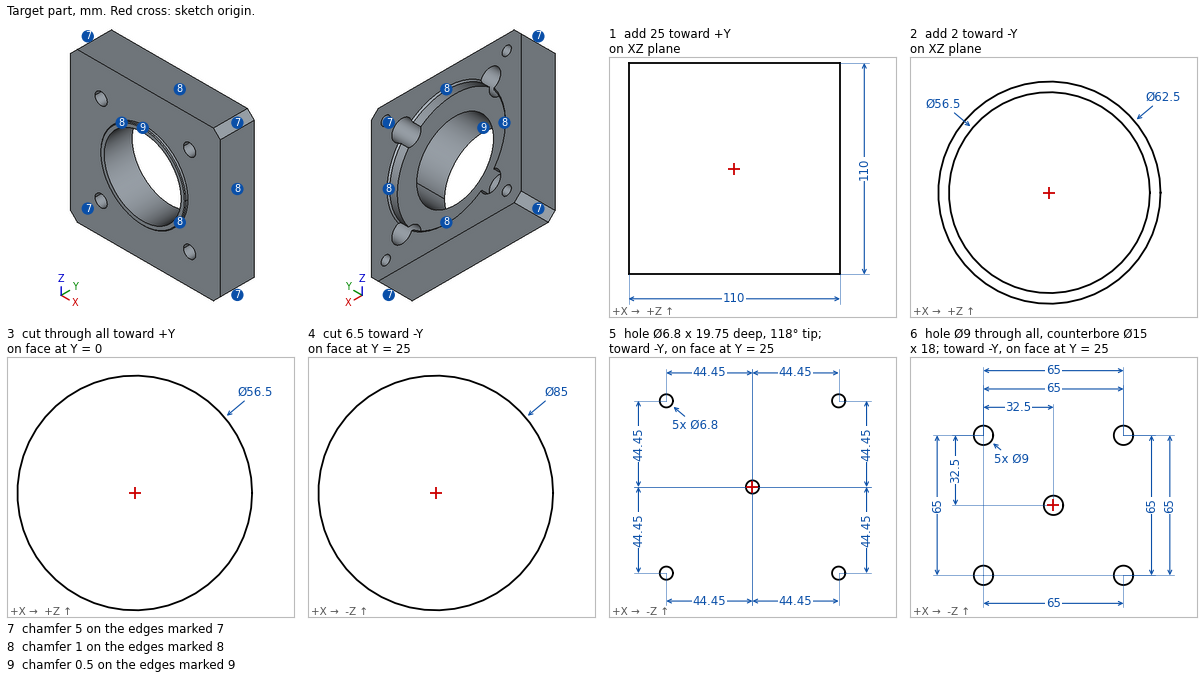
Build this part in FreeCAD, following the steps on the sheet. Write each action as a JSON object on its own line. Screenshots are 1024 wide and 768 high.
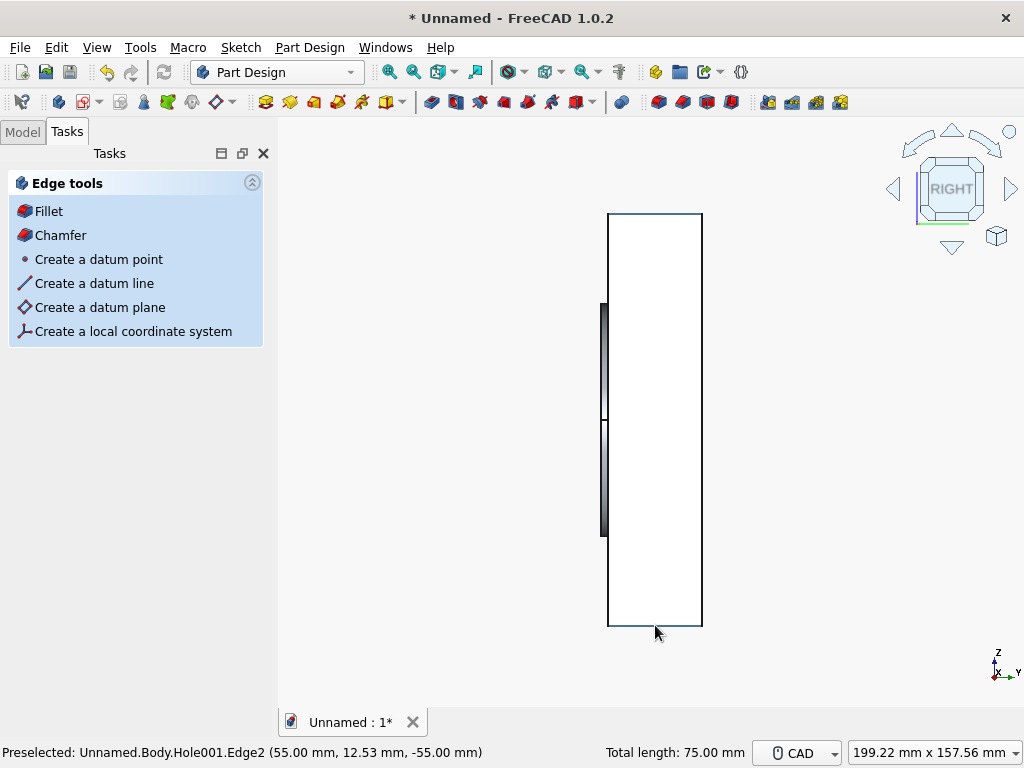
{"action": "key", "text": "5"}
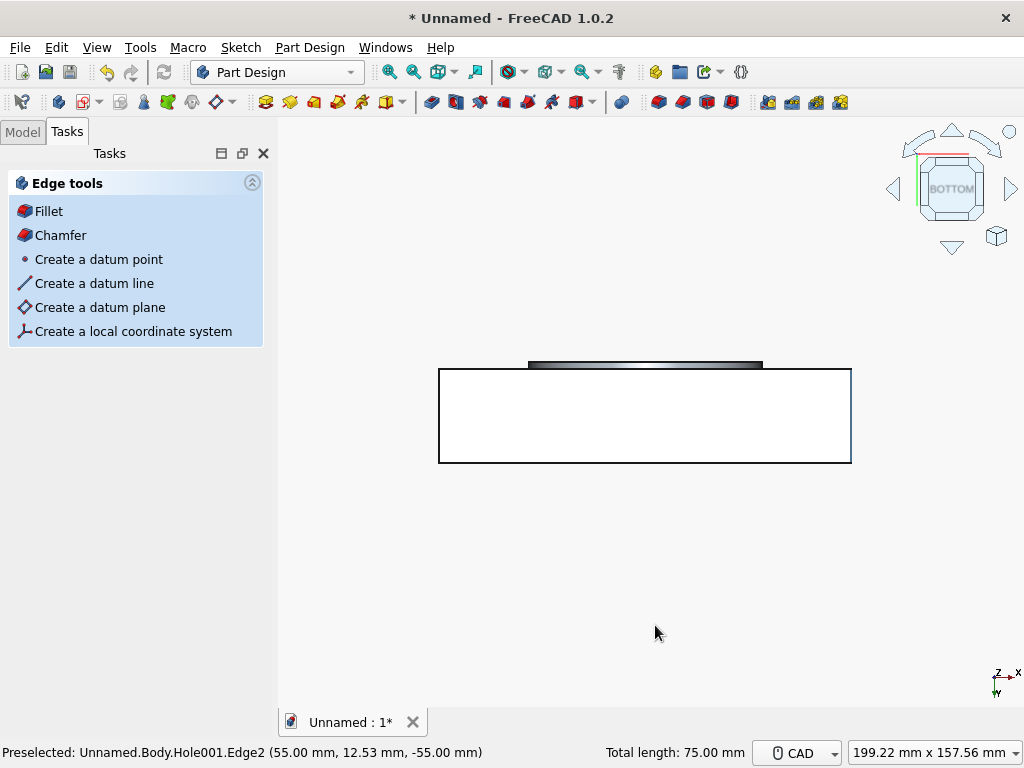
{"action": "left_click", "coordinate": [439, 415], "text": "ctrl"}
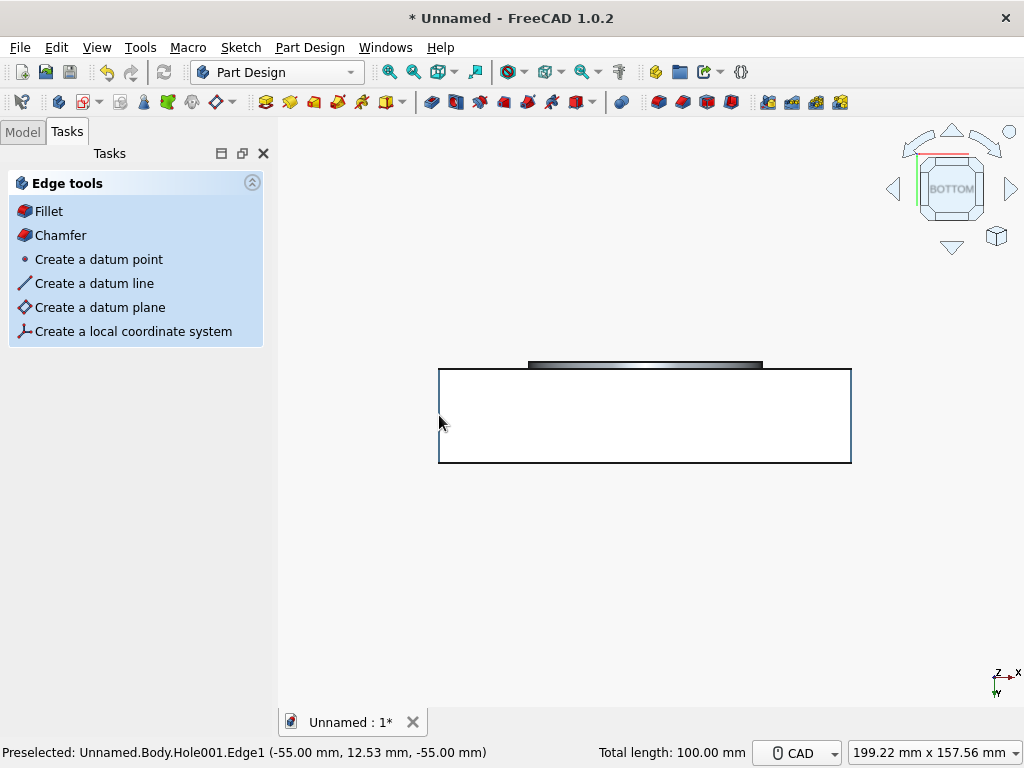
{"action": "left_click", "coordinate": [684, 102]}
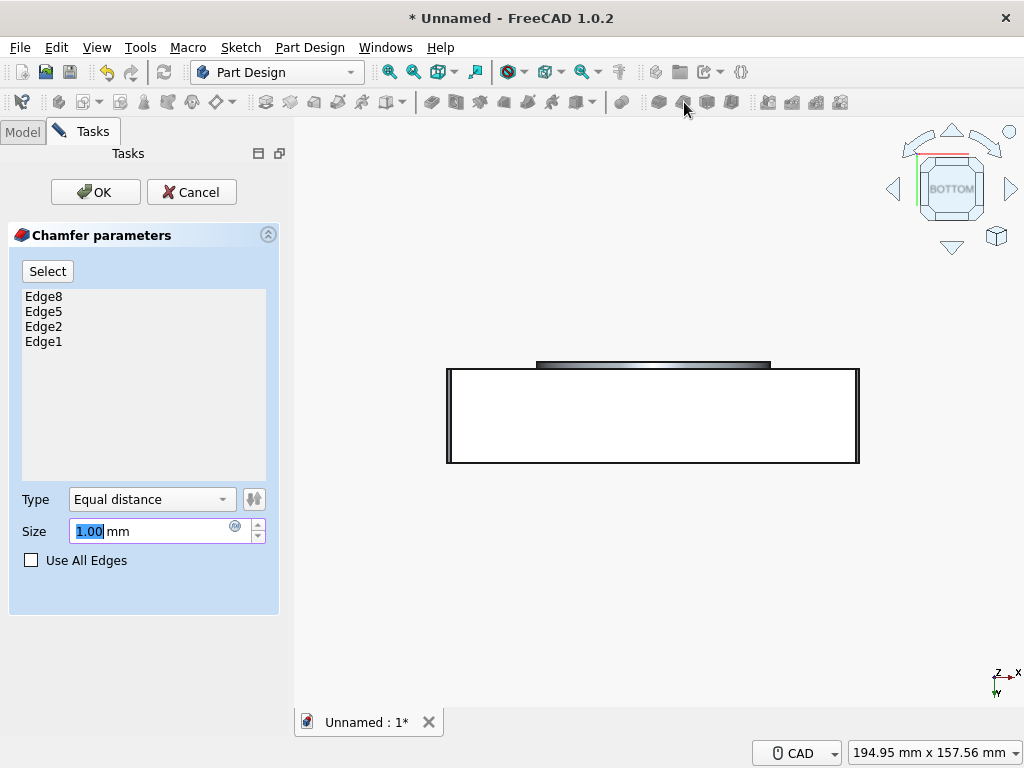
{"action": "type", "text": "5"}
{"action": "key", "text": "Tab"}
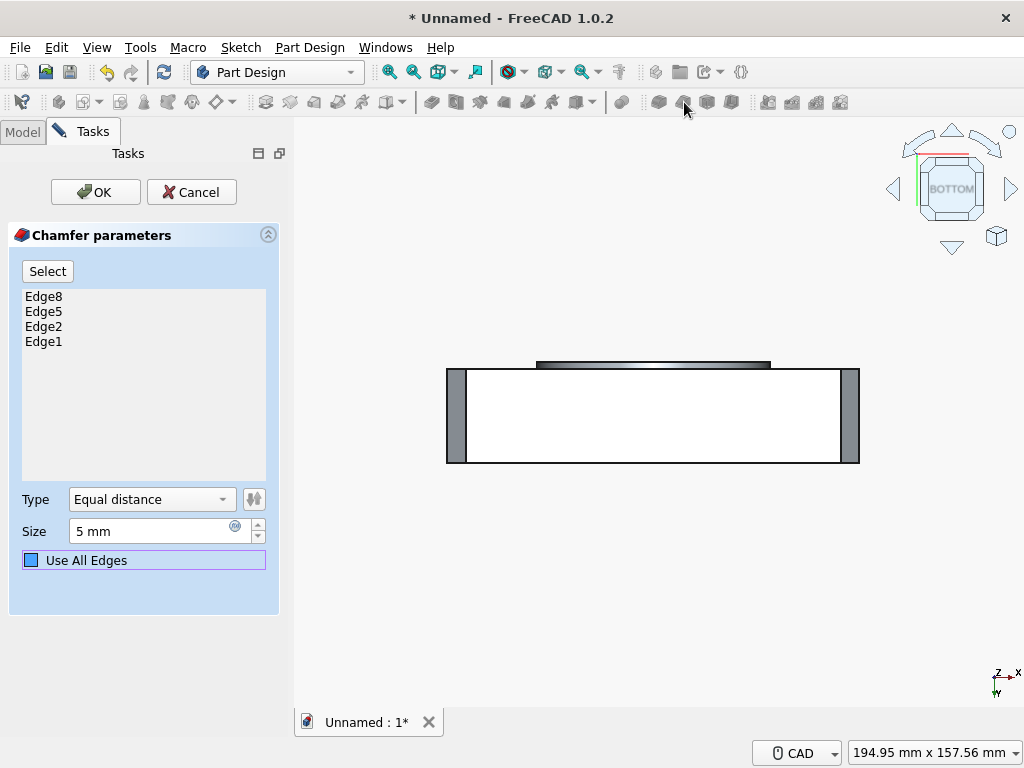
{"action": "left_click", "coordinate": [96, 192]}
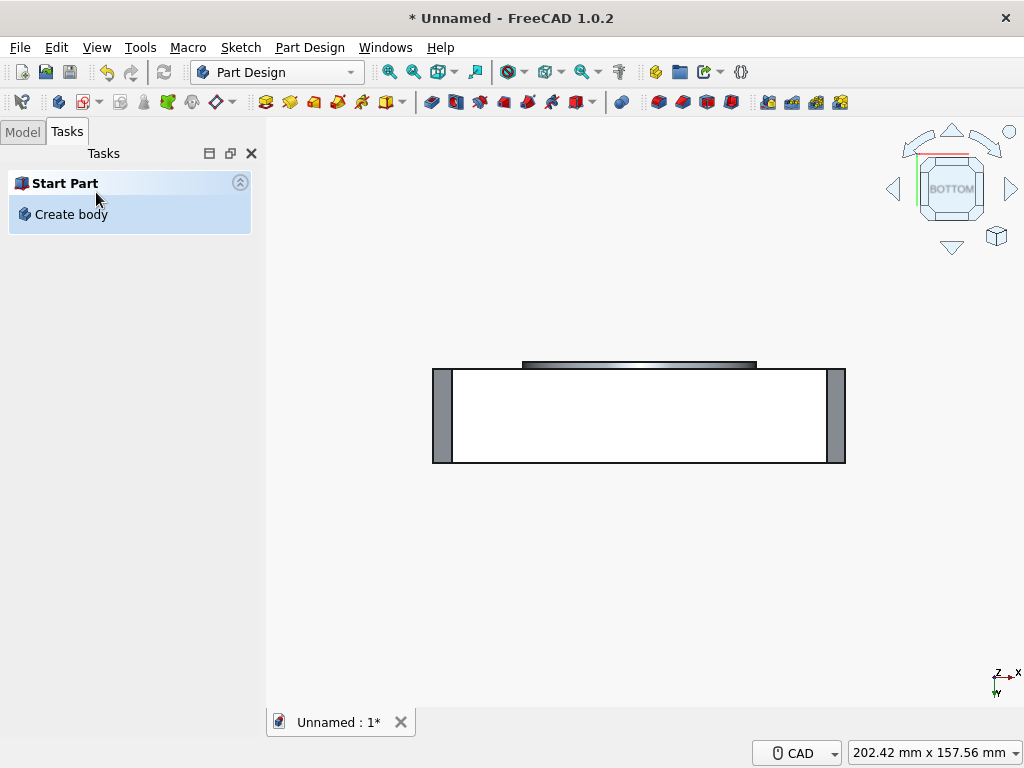
{"action": "key", "text": "0"}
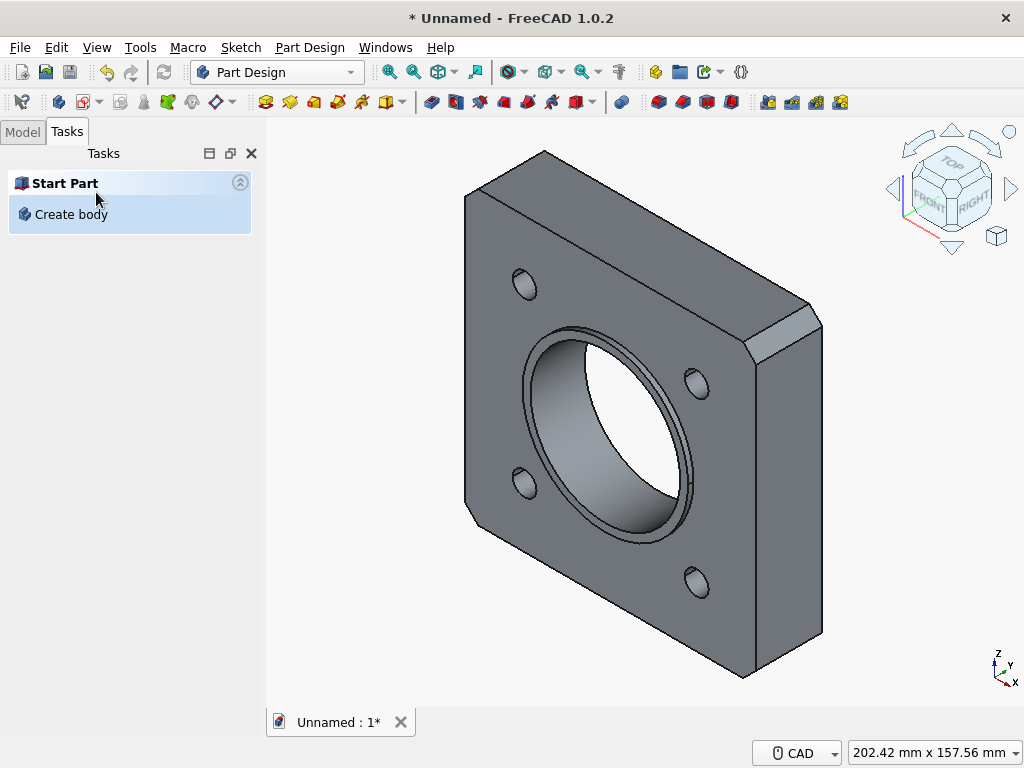
{"action": "key", "text": "2"}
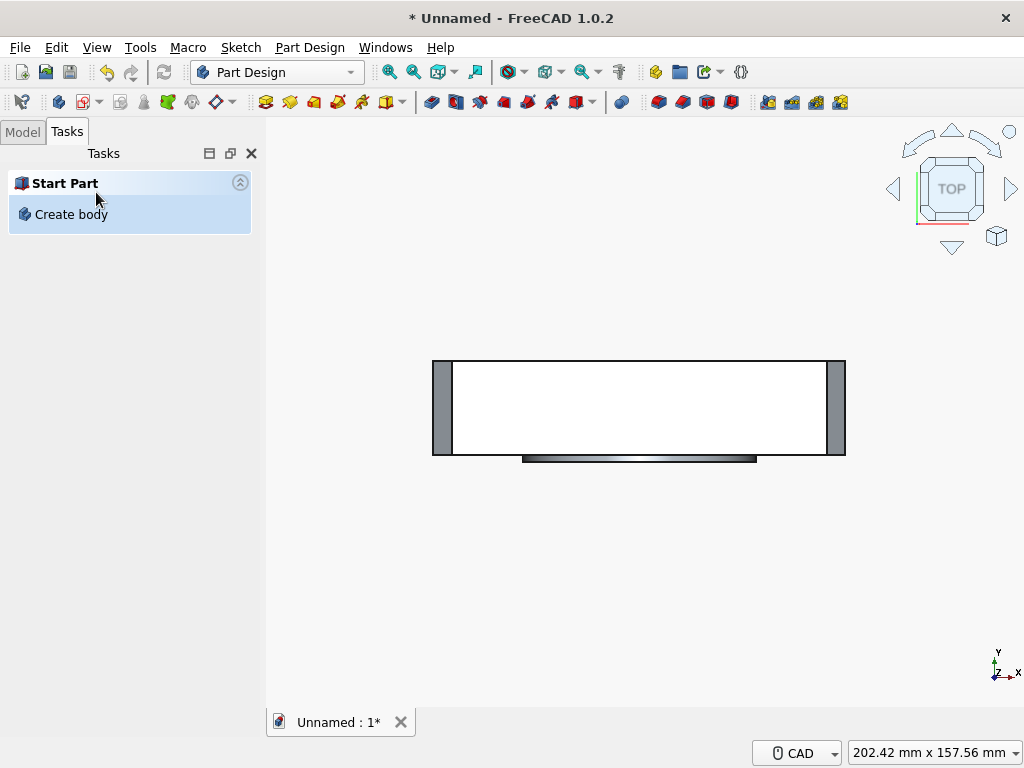
{"action": "key", "text": "1"}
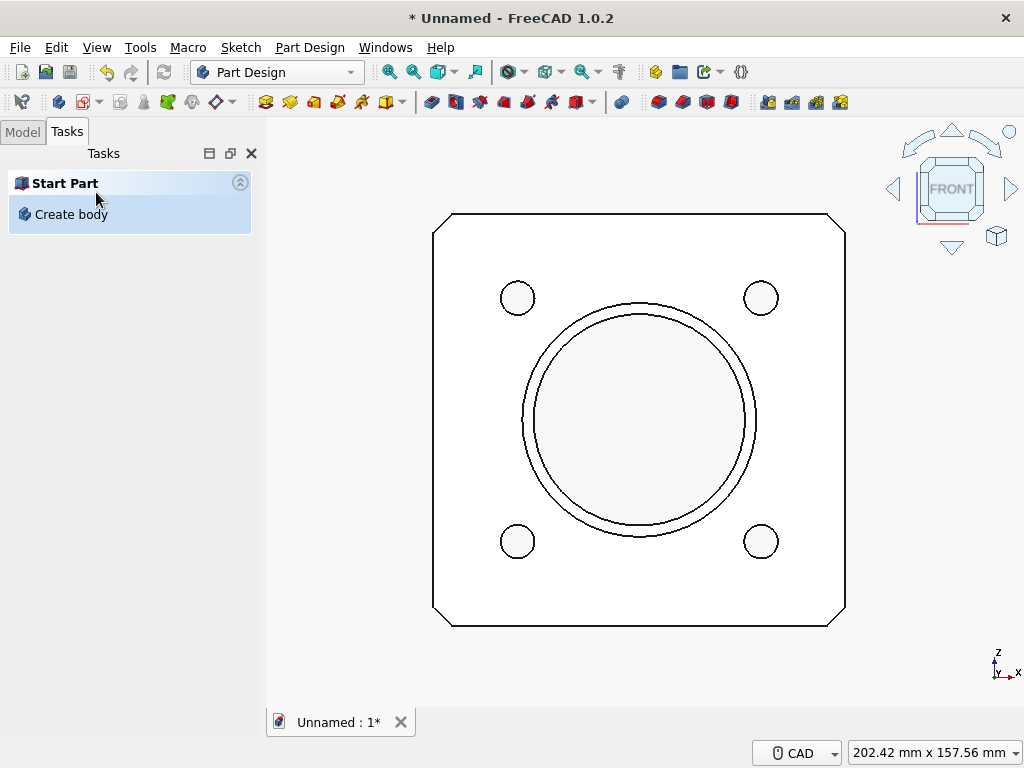
{"action": "key", "text": "3"}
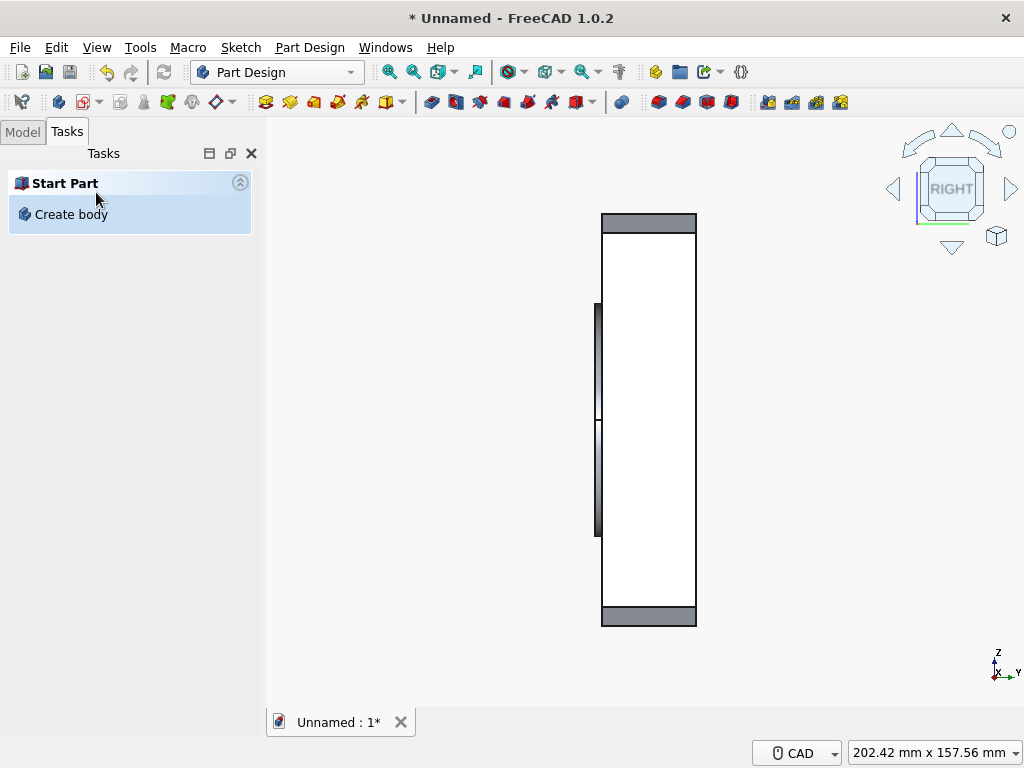
{"action": "key", "text": "5"}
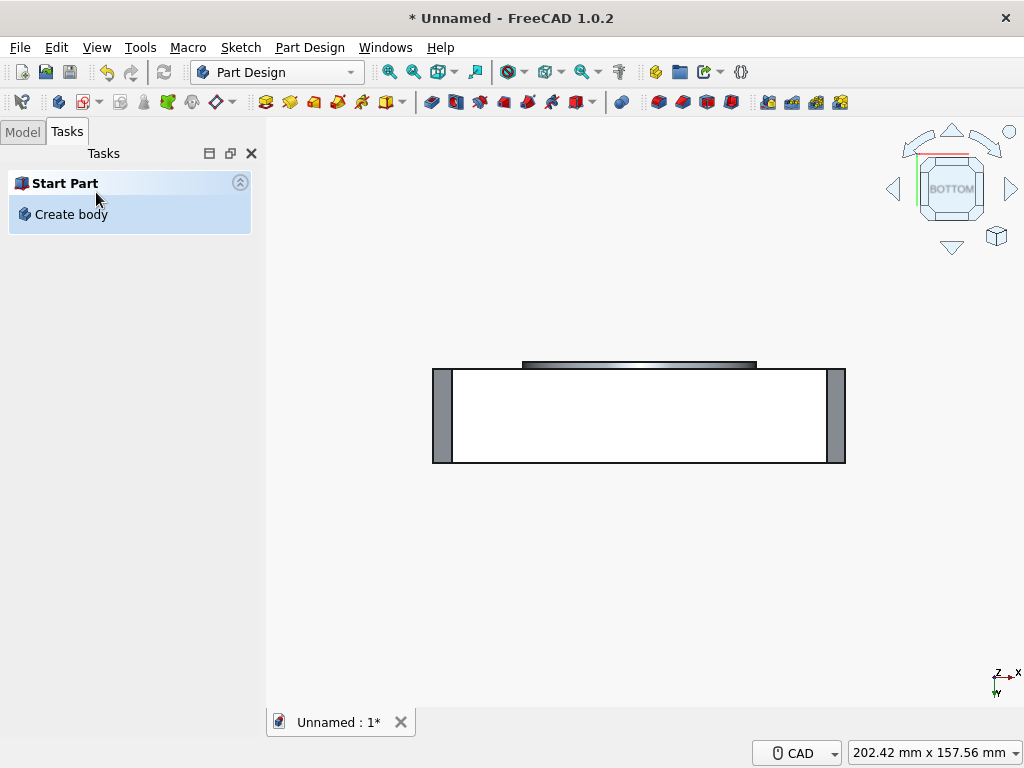
{"action": "key", "text": "4"}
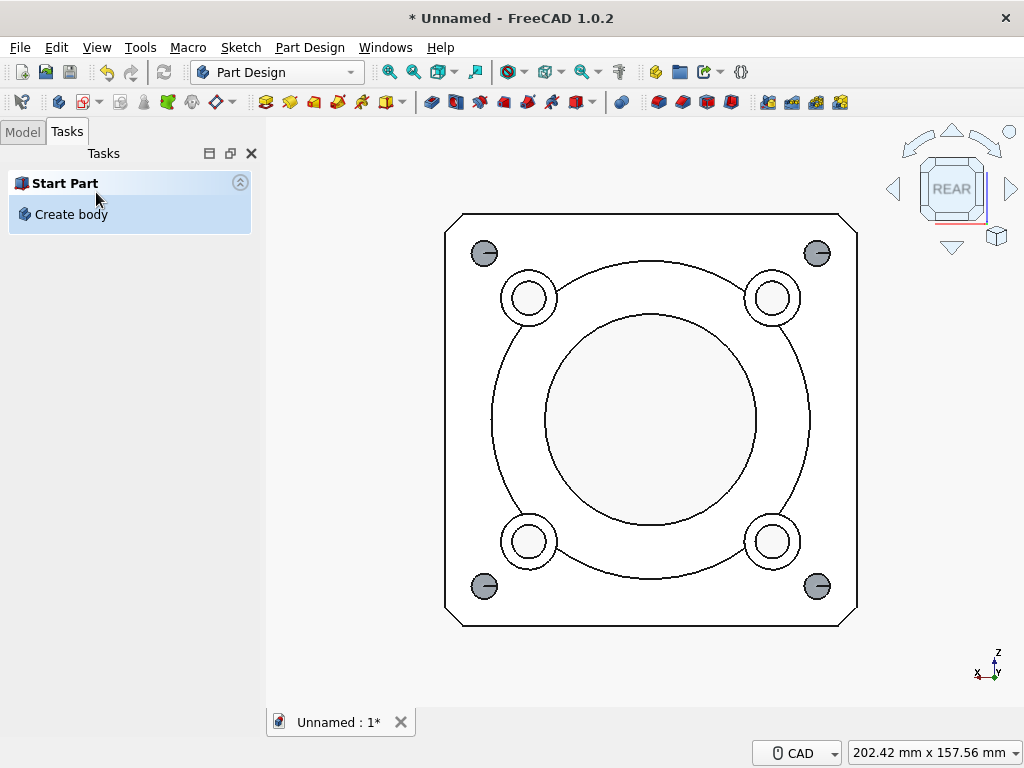
{"action": "left_click", "coordinate": [810, 419]}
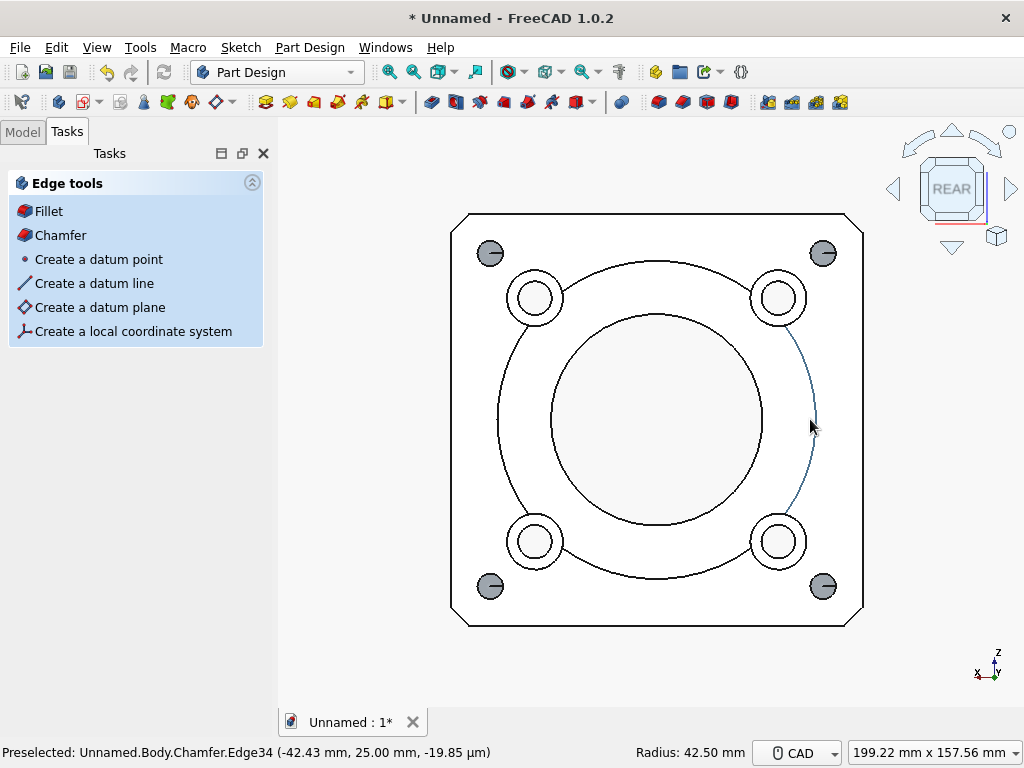
{"action": "left_click", "coordinate": [500, 449], "text": "ctrl"}